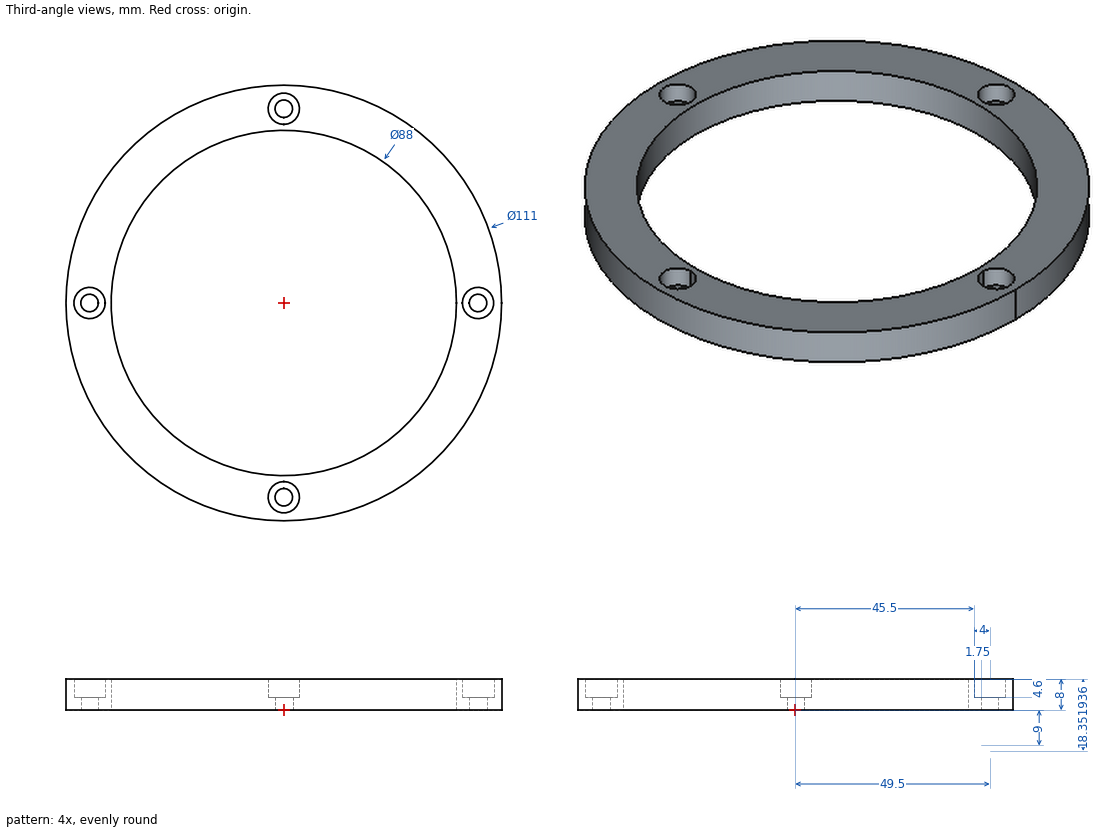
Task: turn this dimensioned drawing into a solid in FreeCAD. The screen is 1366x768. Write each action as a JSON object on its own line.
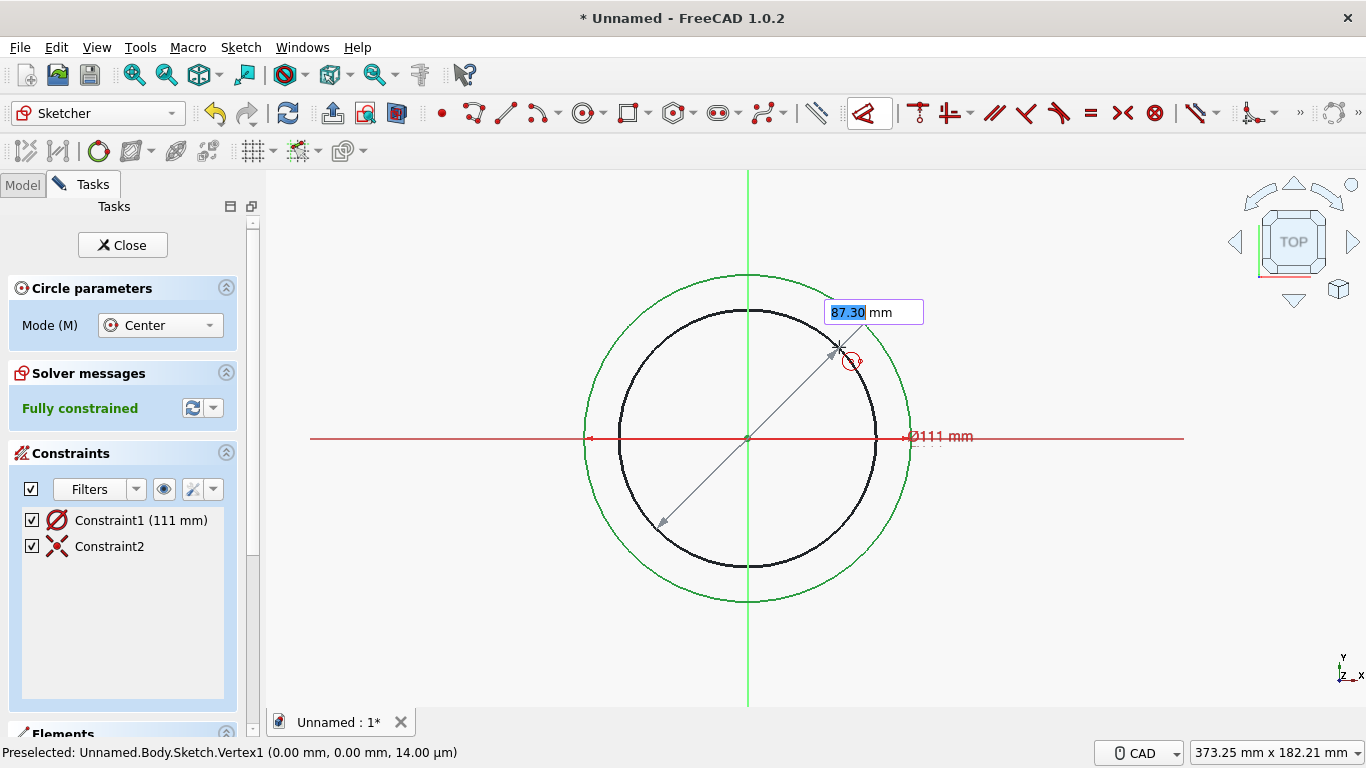
{"action": "type", "text": "88"}
{"action": "key", "text": "Return"}
{"action": "key", "text": "Escape"}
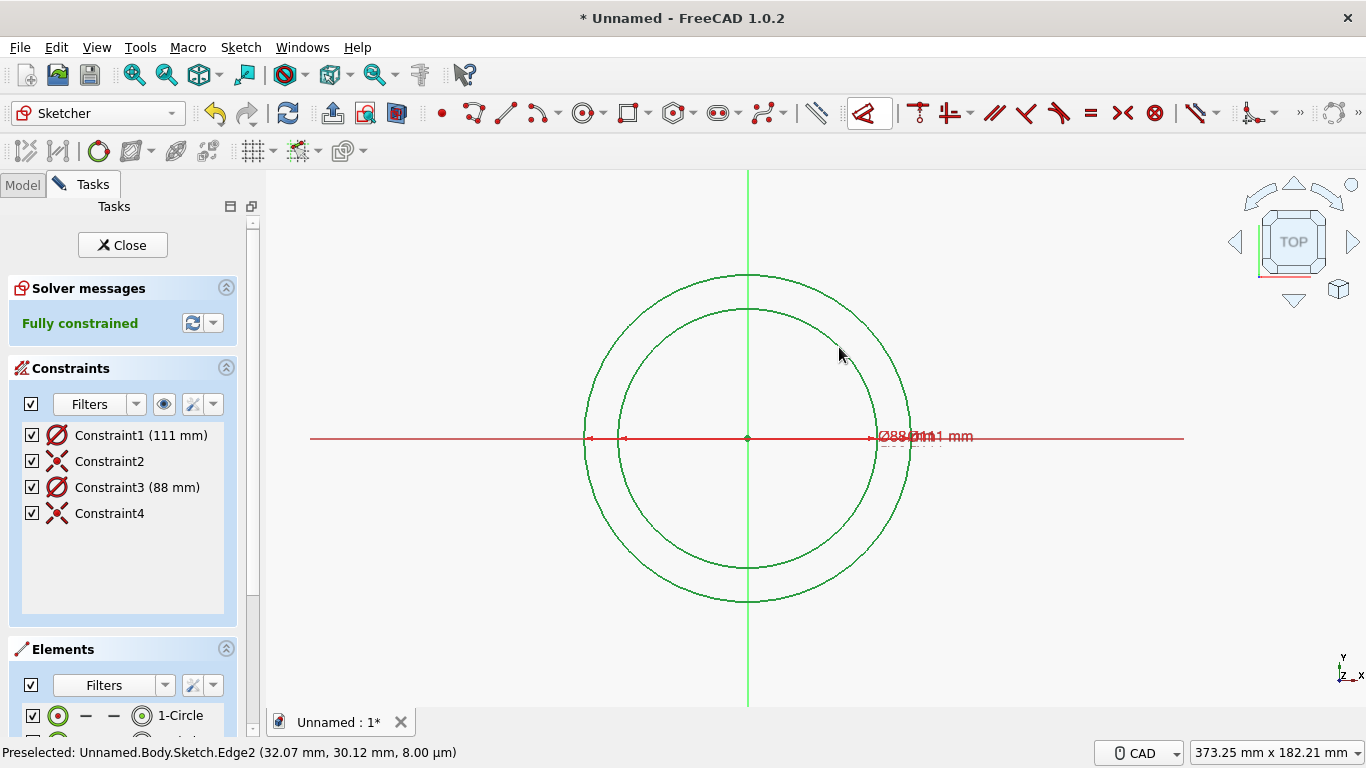
{"action": "left_click", "coordinate": [123, 245]}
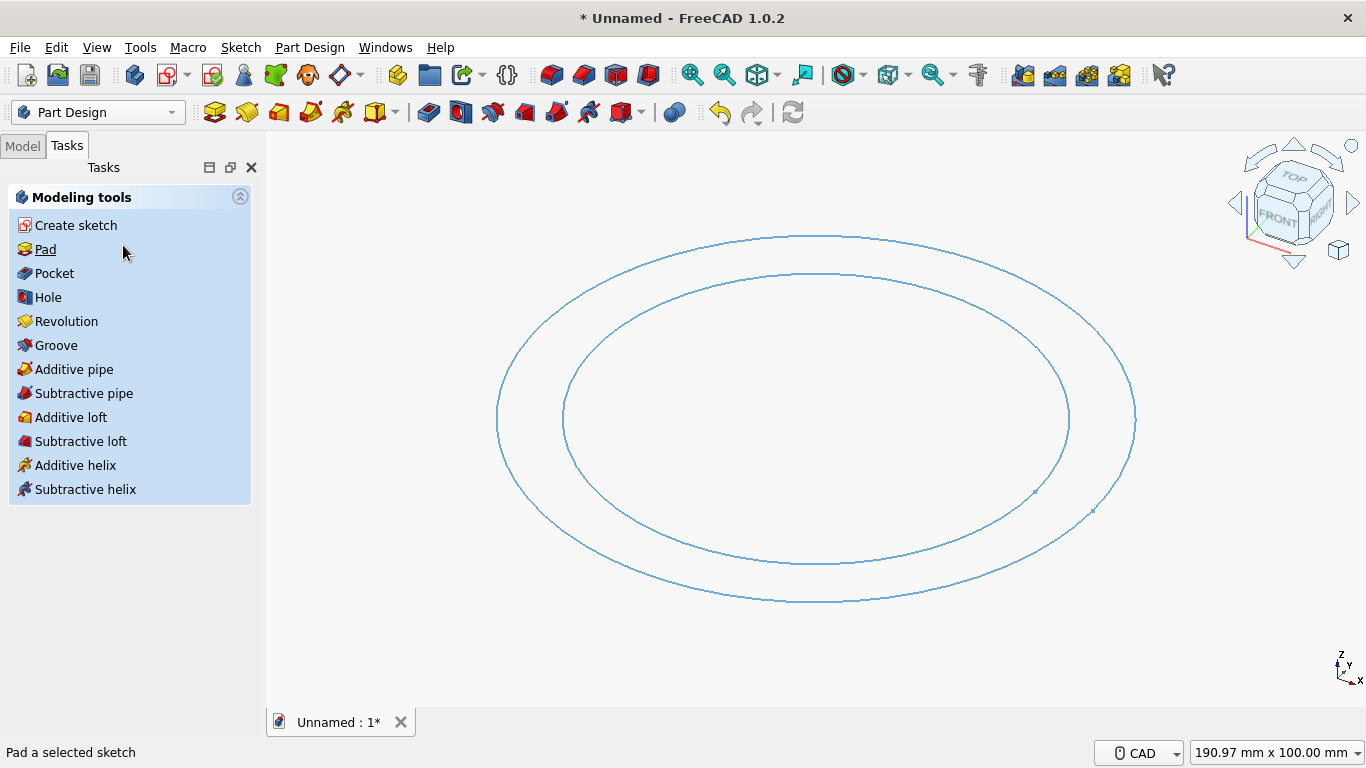
{"action": "left_click", "coordinate": [216, 112]}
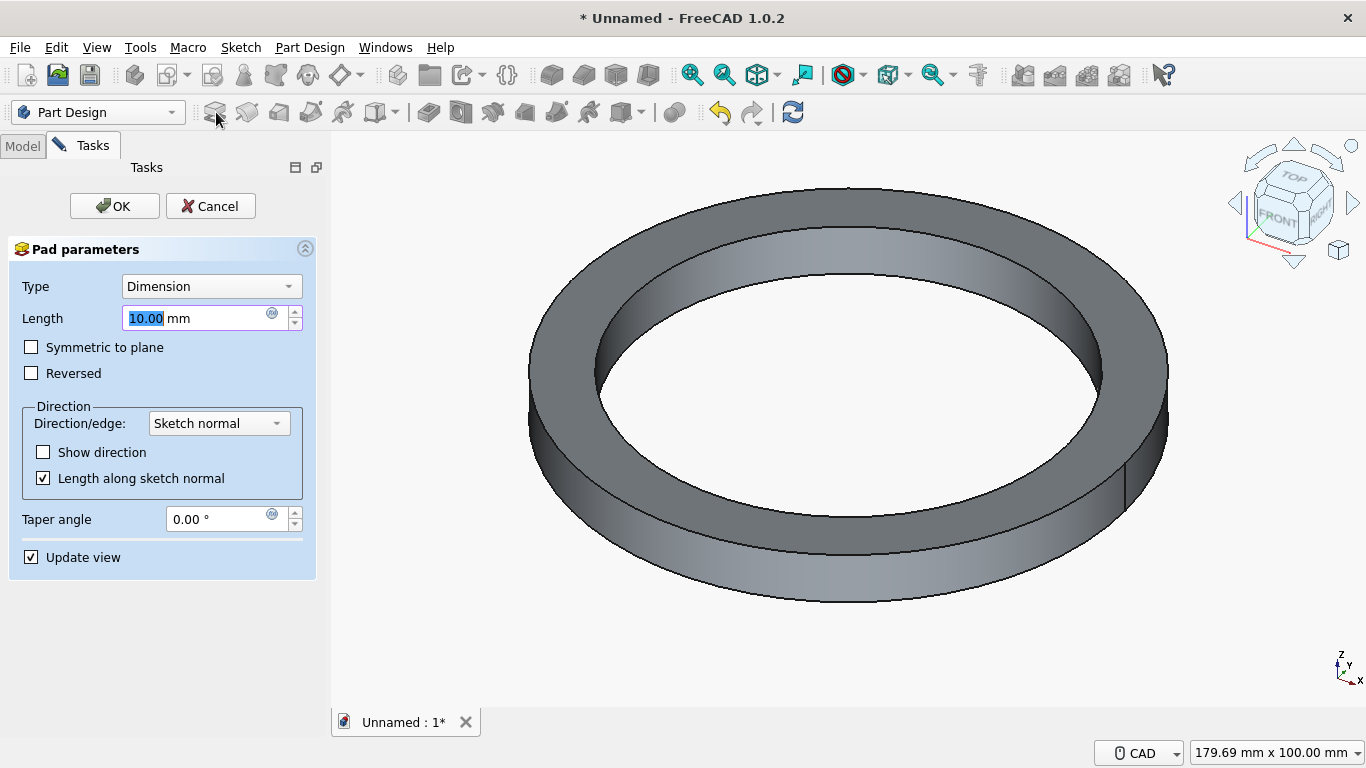
{"action": "type", "text": "8"}
{"action": "key", "text": "Tab"}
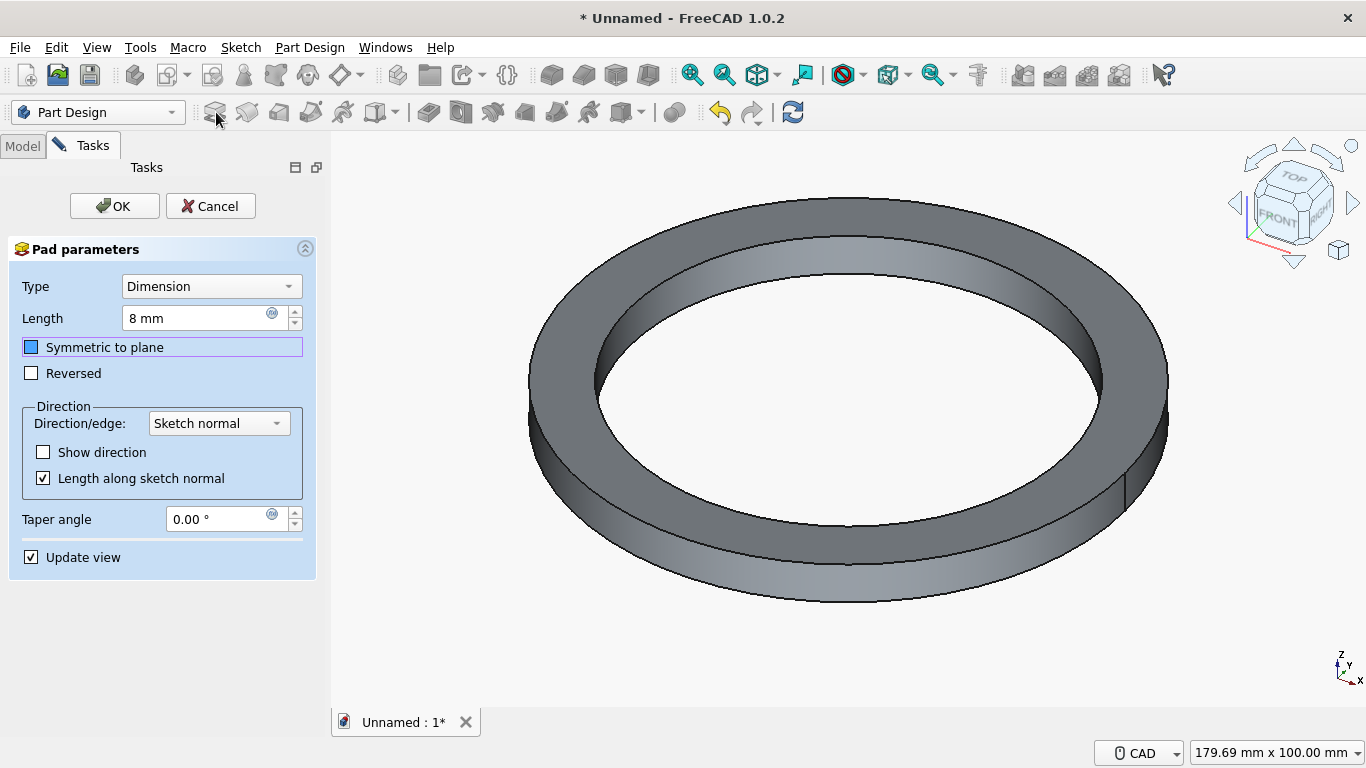
{"action": "left_click", "coordinate": [115, 206]}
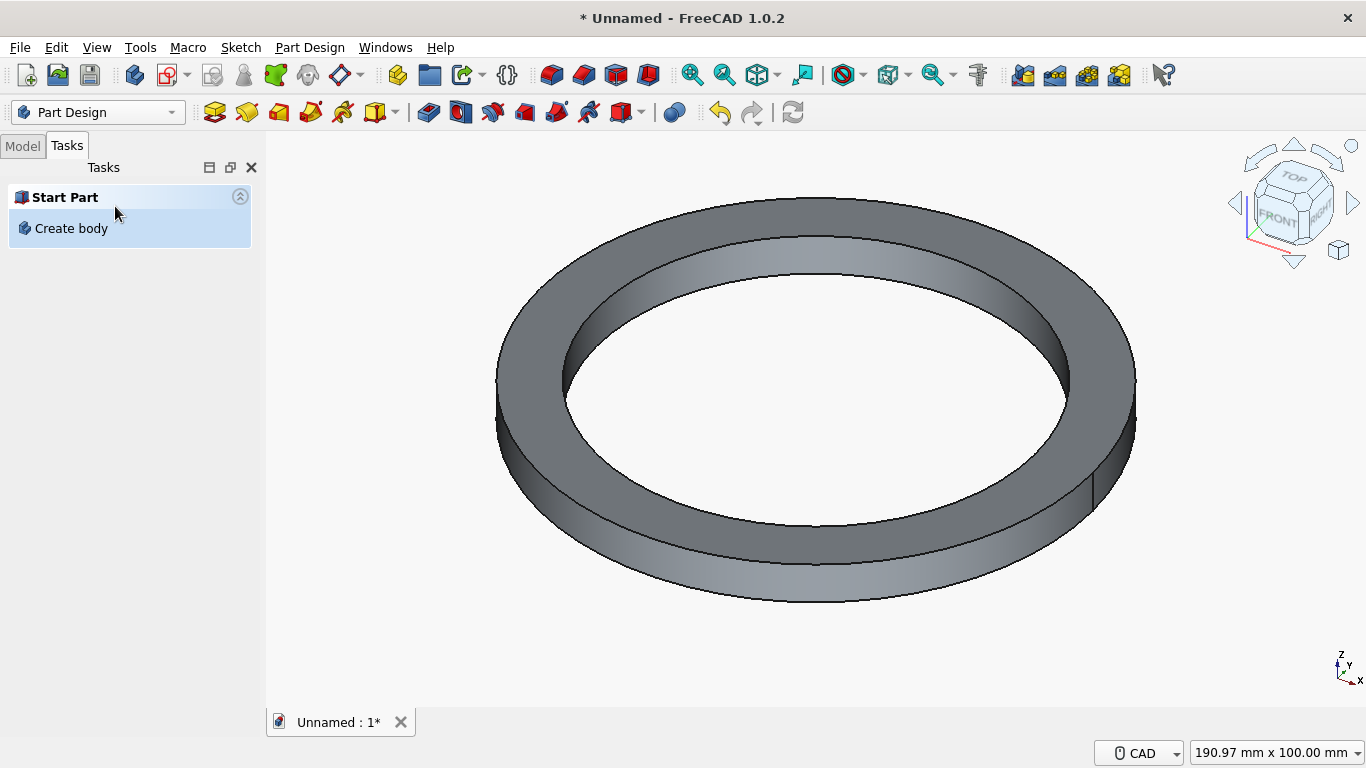
{"action": "key", "text": "v f"}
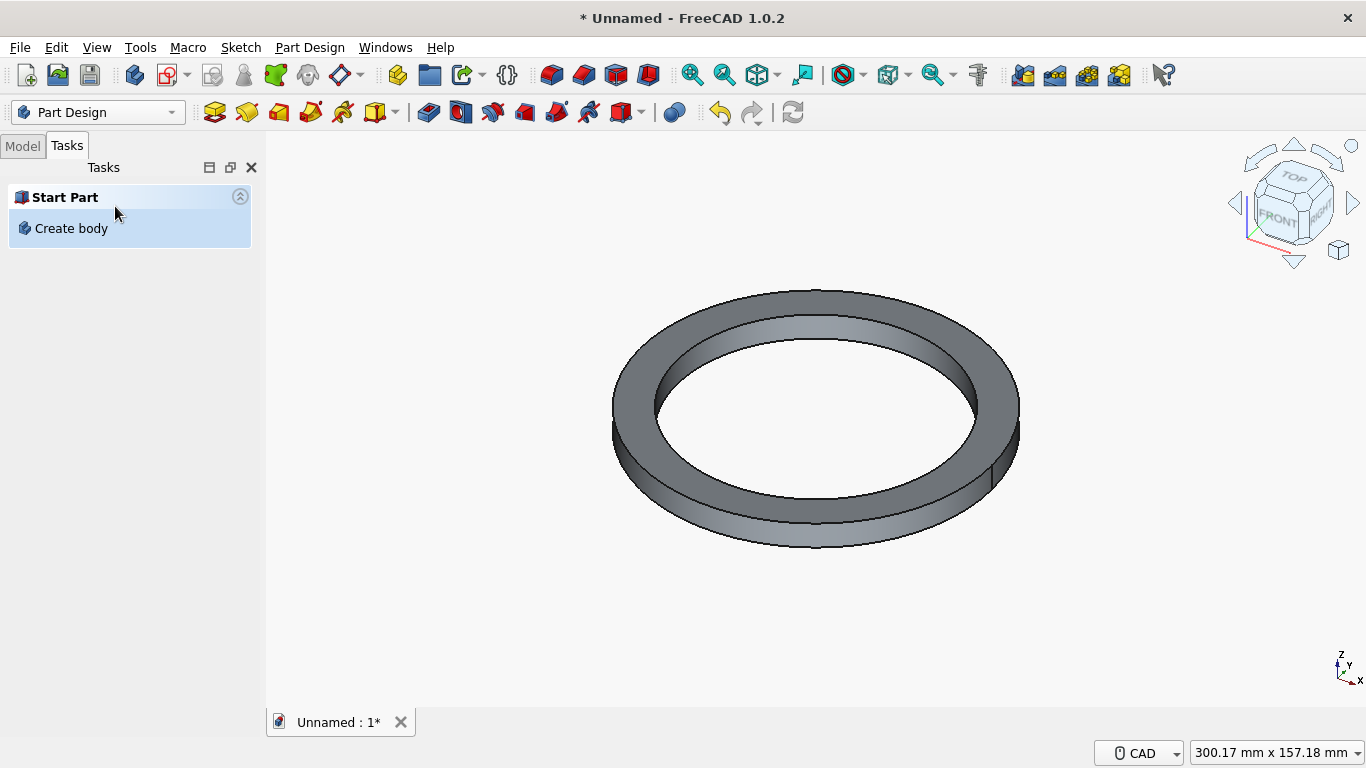
{"action": "left_click", "coordinate": [168, 76]}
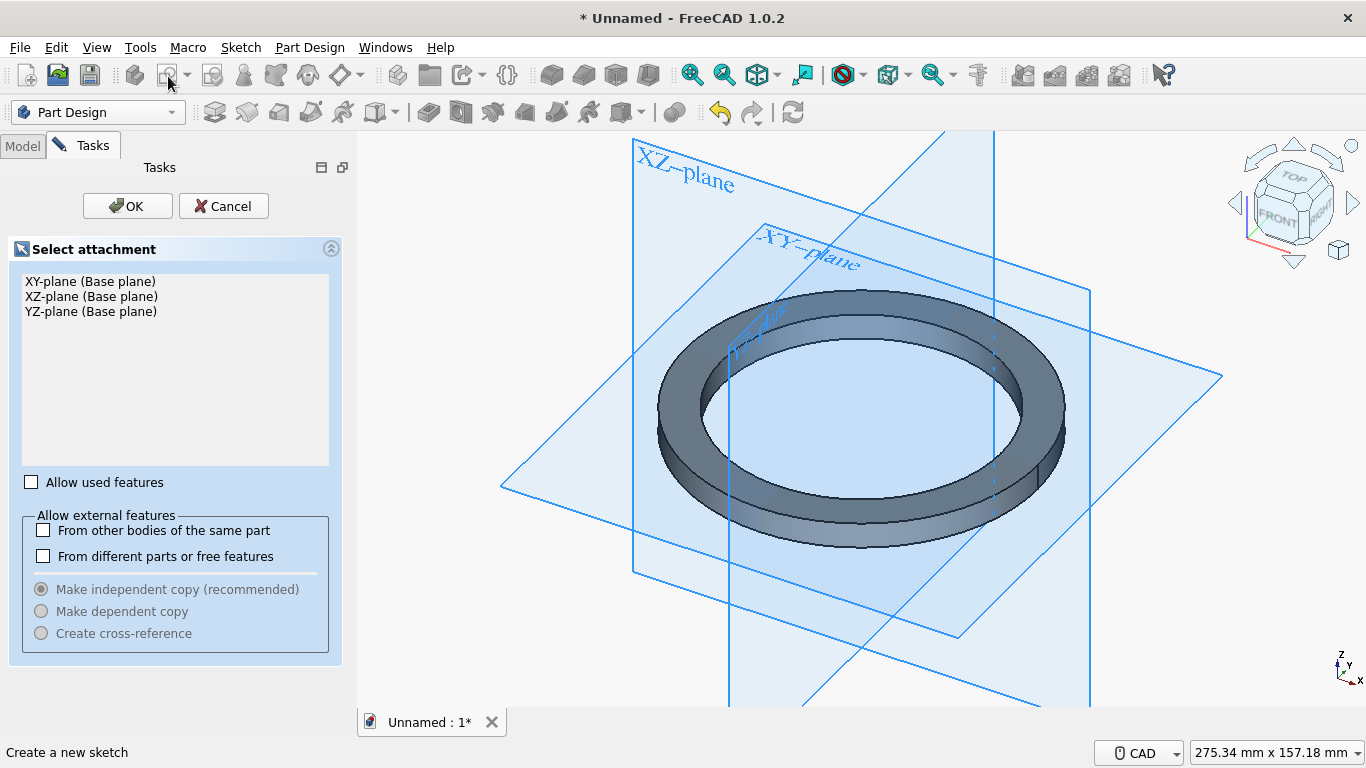
{"action": "left_click", "coordinate": [82, 312]}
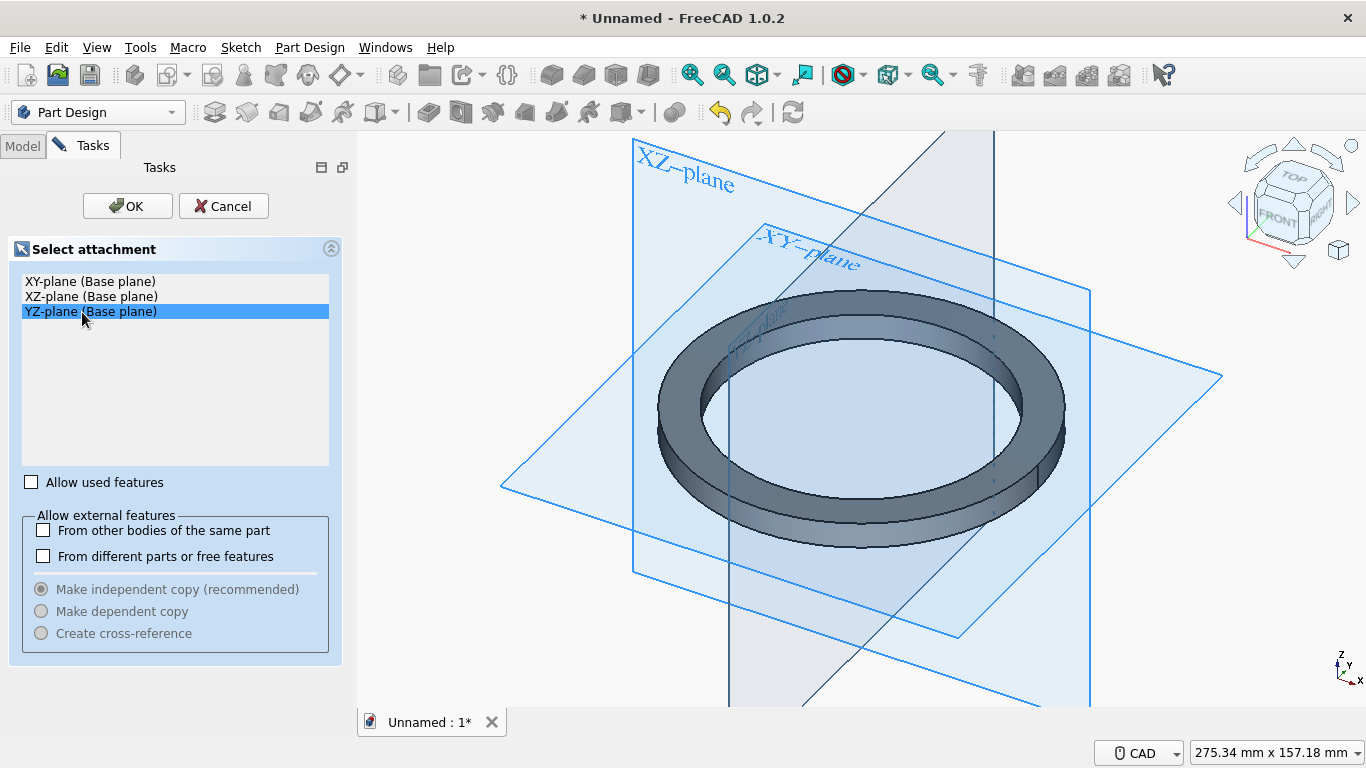
{"action": "left_click", "coordinate": [128, 206]}